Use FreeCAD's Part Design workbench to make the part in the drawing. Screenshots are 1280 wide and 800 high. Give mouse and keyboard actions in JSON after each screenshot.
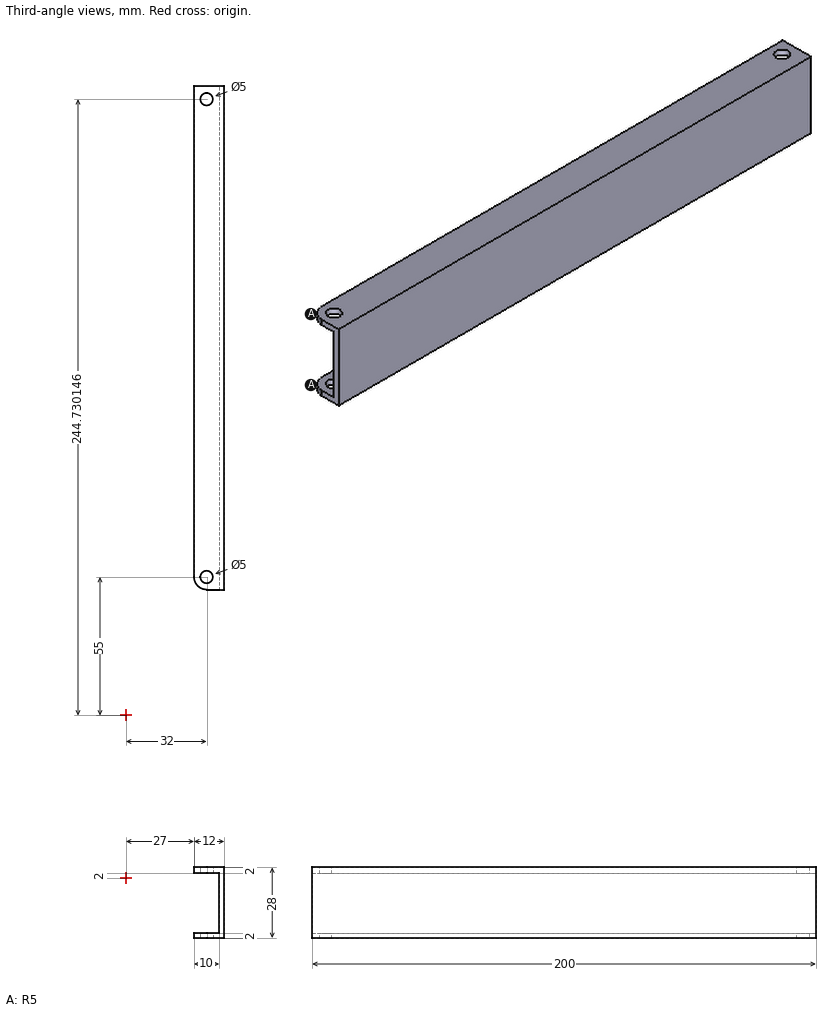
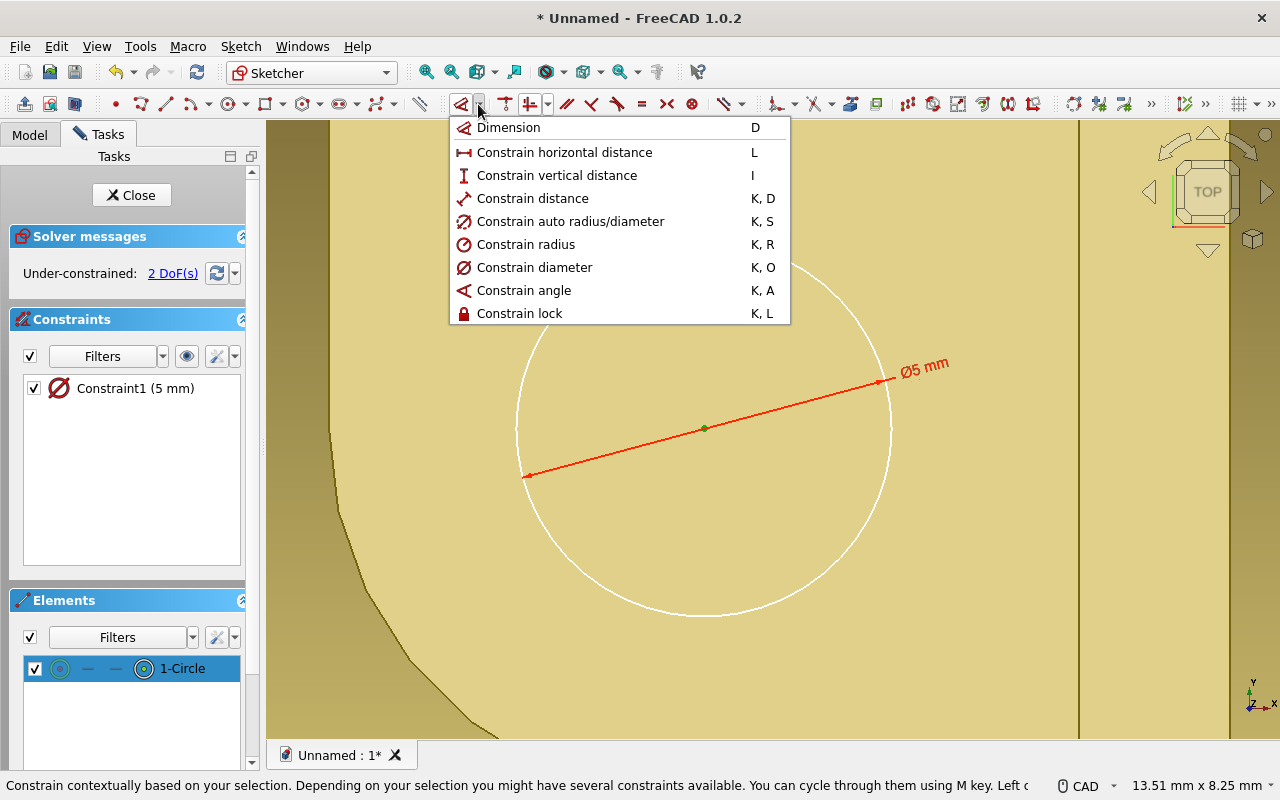
{"action": "left_click", "coordinate": [620, 152]}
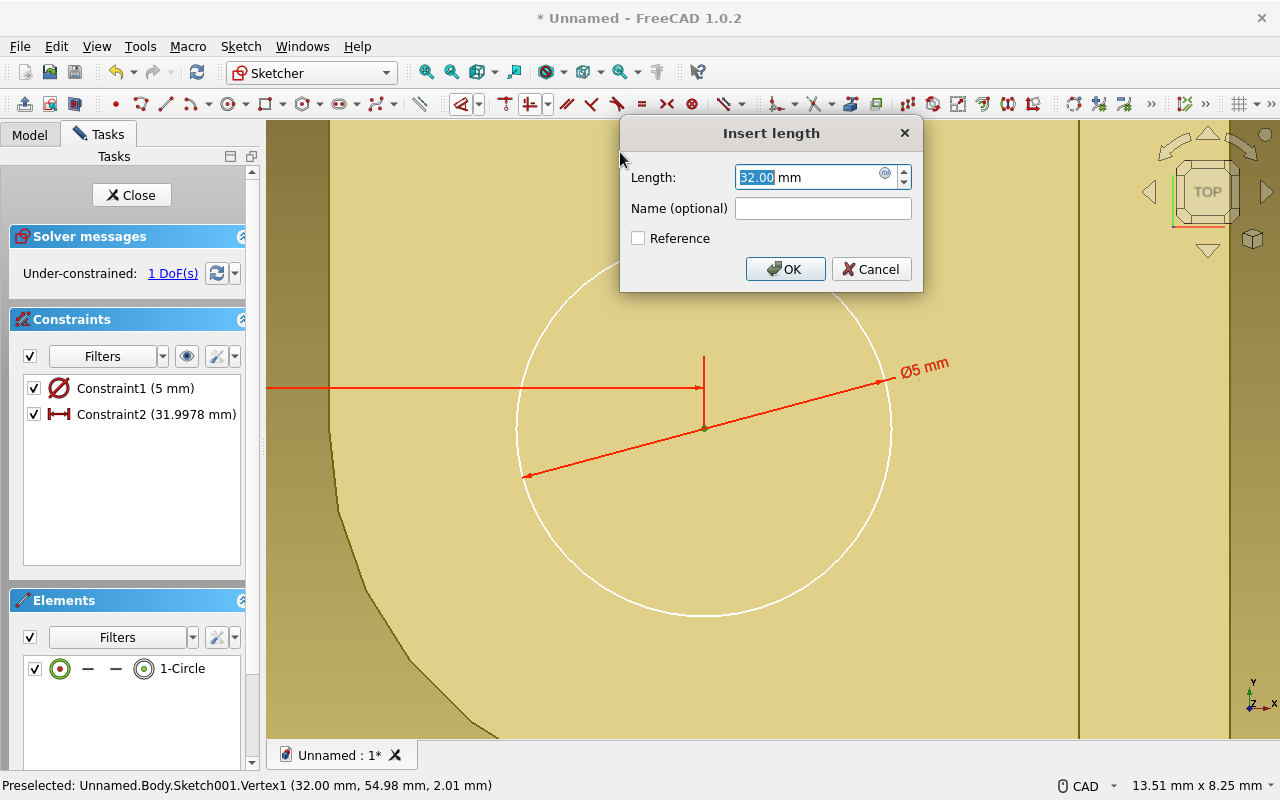
{"action": "type", "text": "32"}
{"action": "key", "text": "Return"}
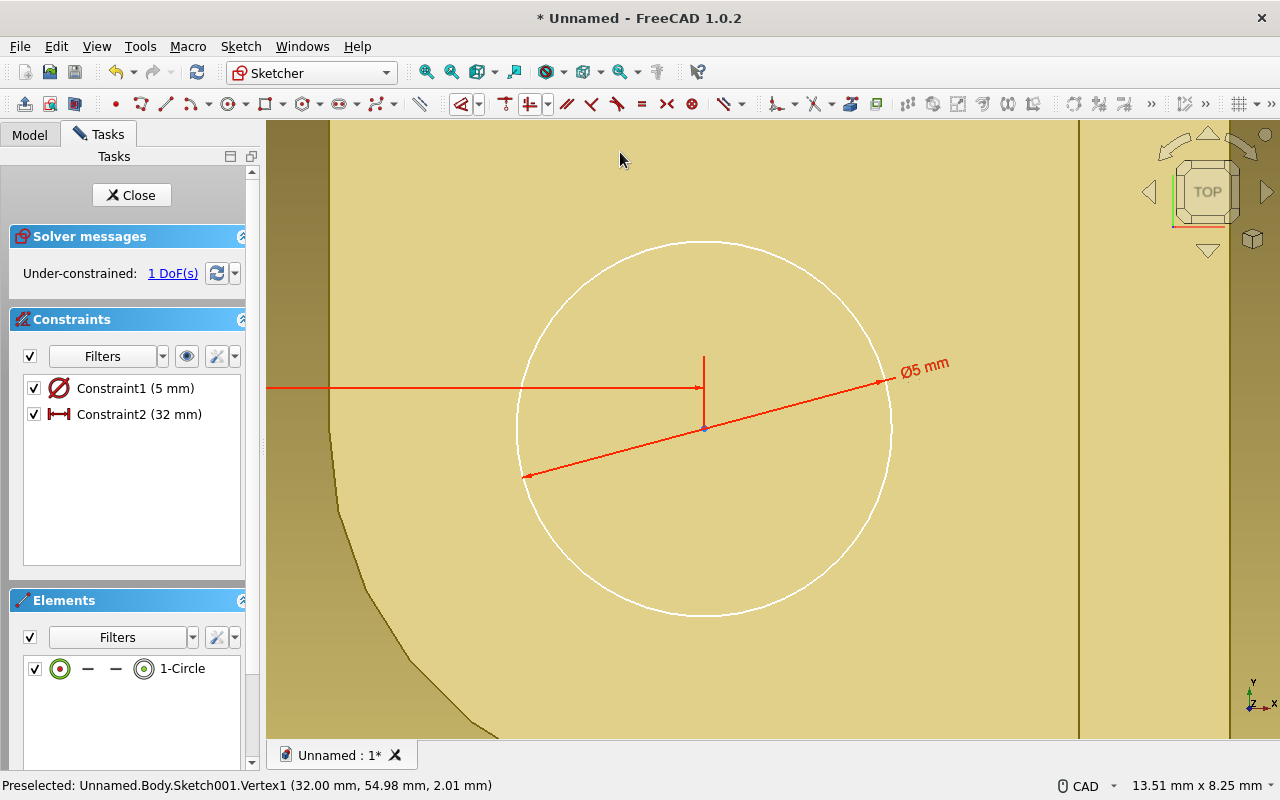
{"action": "left_click", "coordinate": [704, 429]}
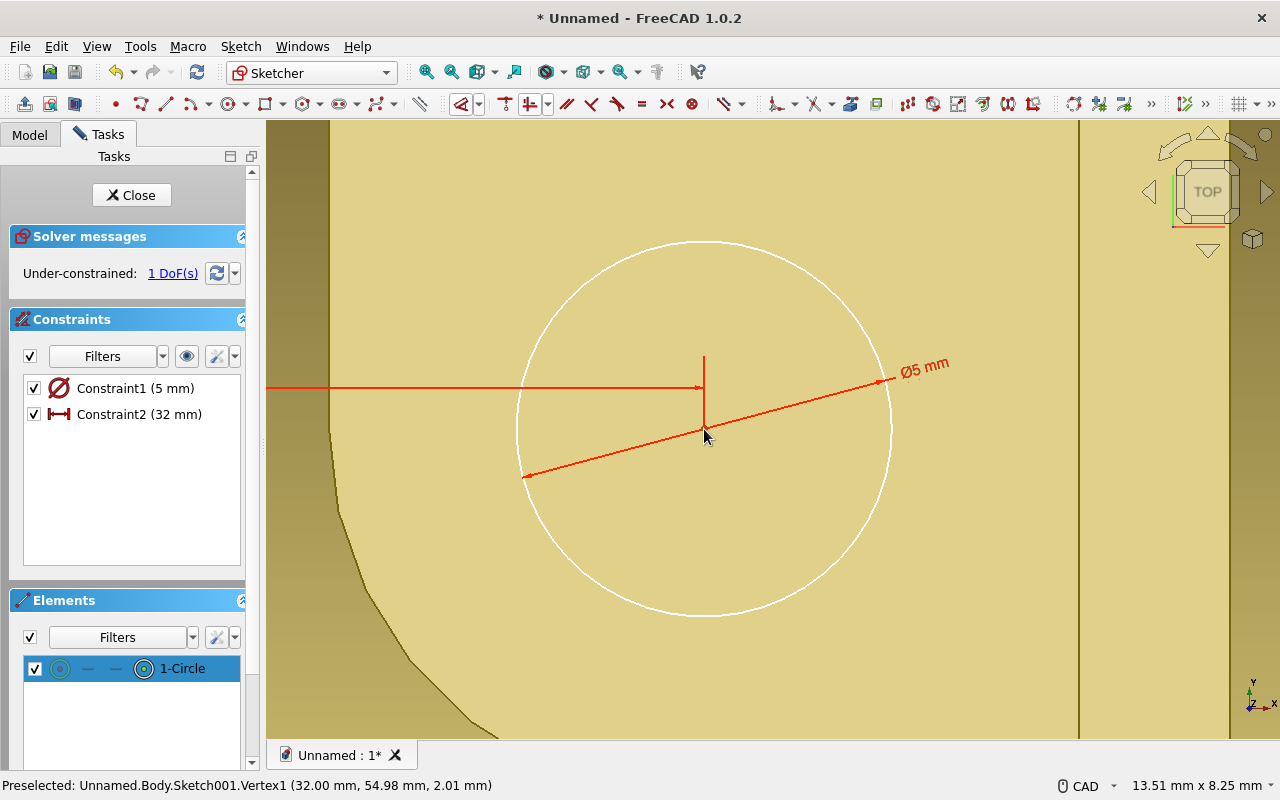
{"action": "key", "text": "i"}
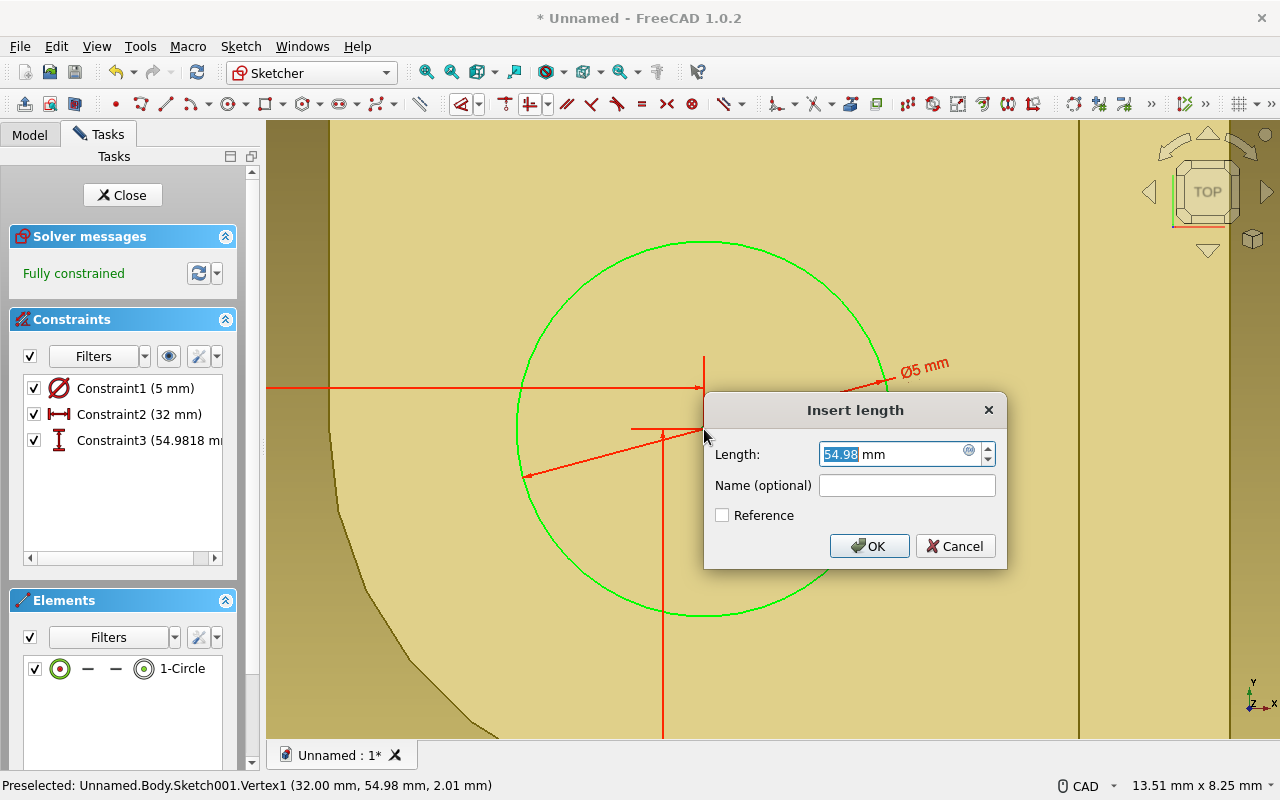
{"action": "type", "text": "55"}
{"action": "key", "text": "Return"}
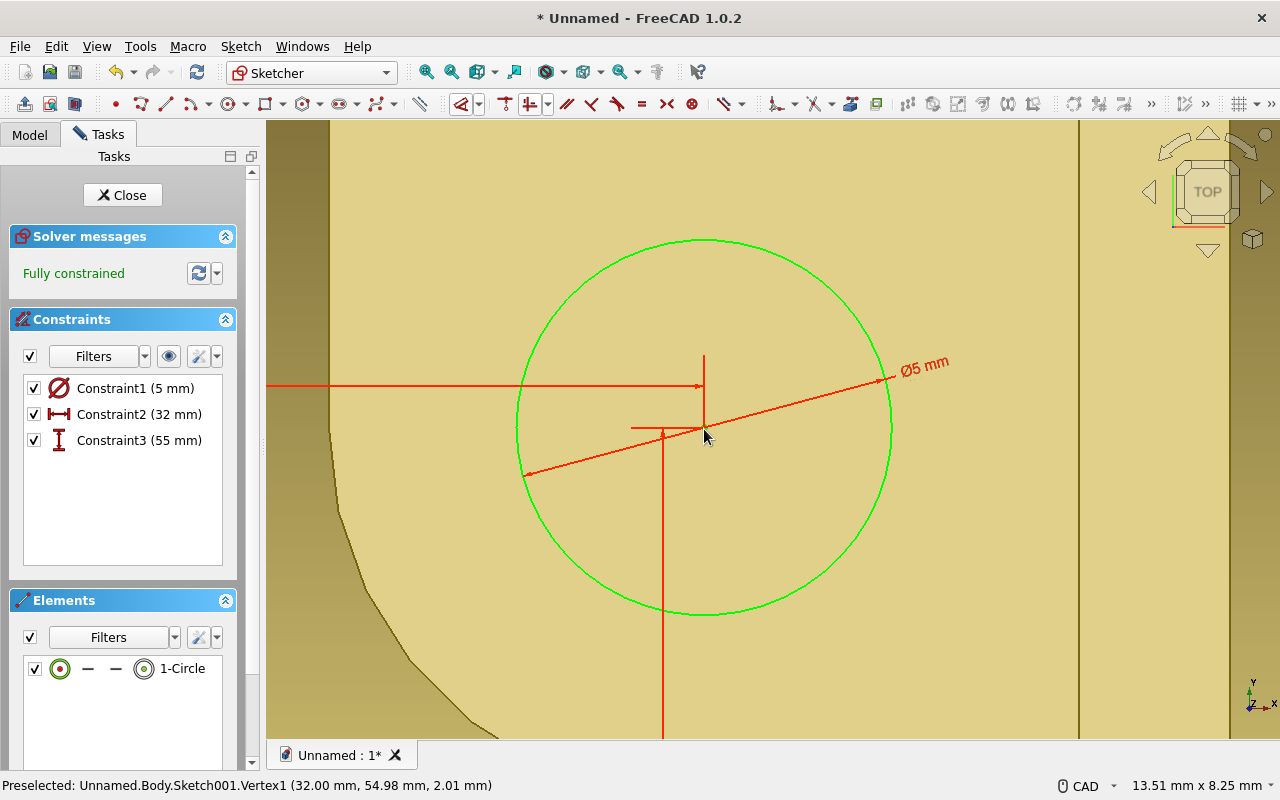
{"action": "left_click", "coordinate": [123, 195]}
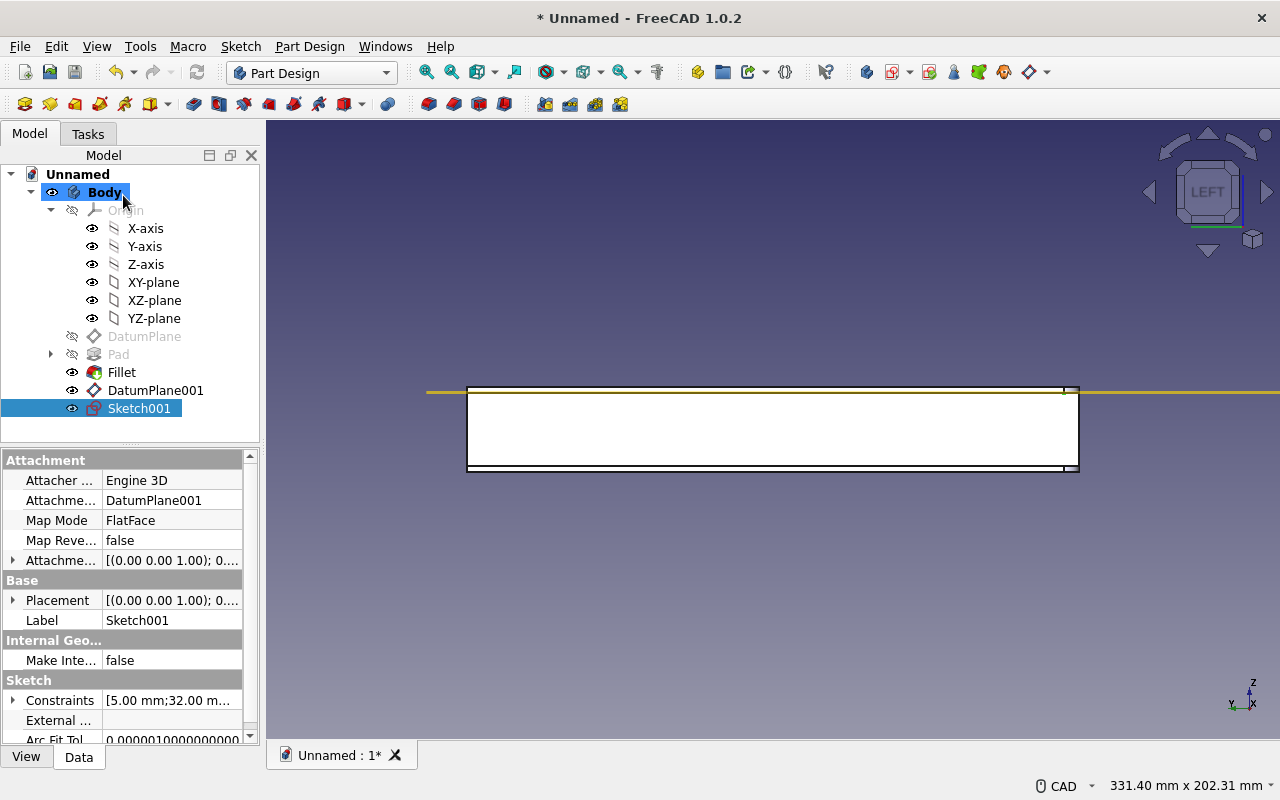
{"action": "left_click", "coordinate": [194, 104]}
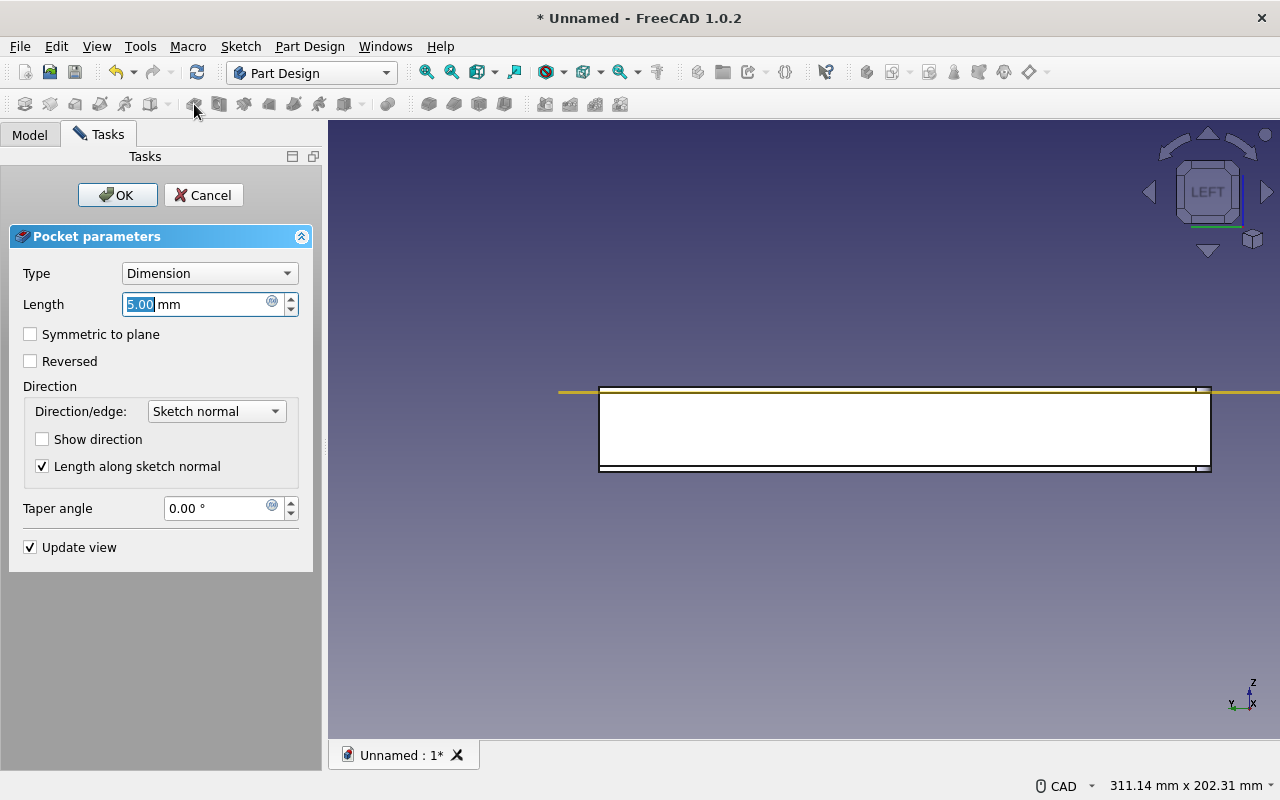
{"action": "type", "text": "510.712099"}
{"action": "key", "text": "Tab"}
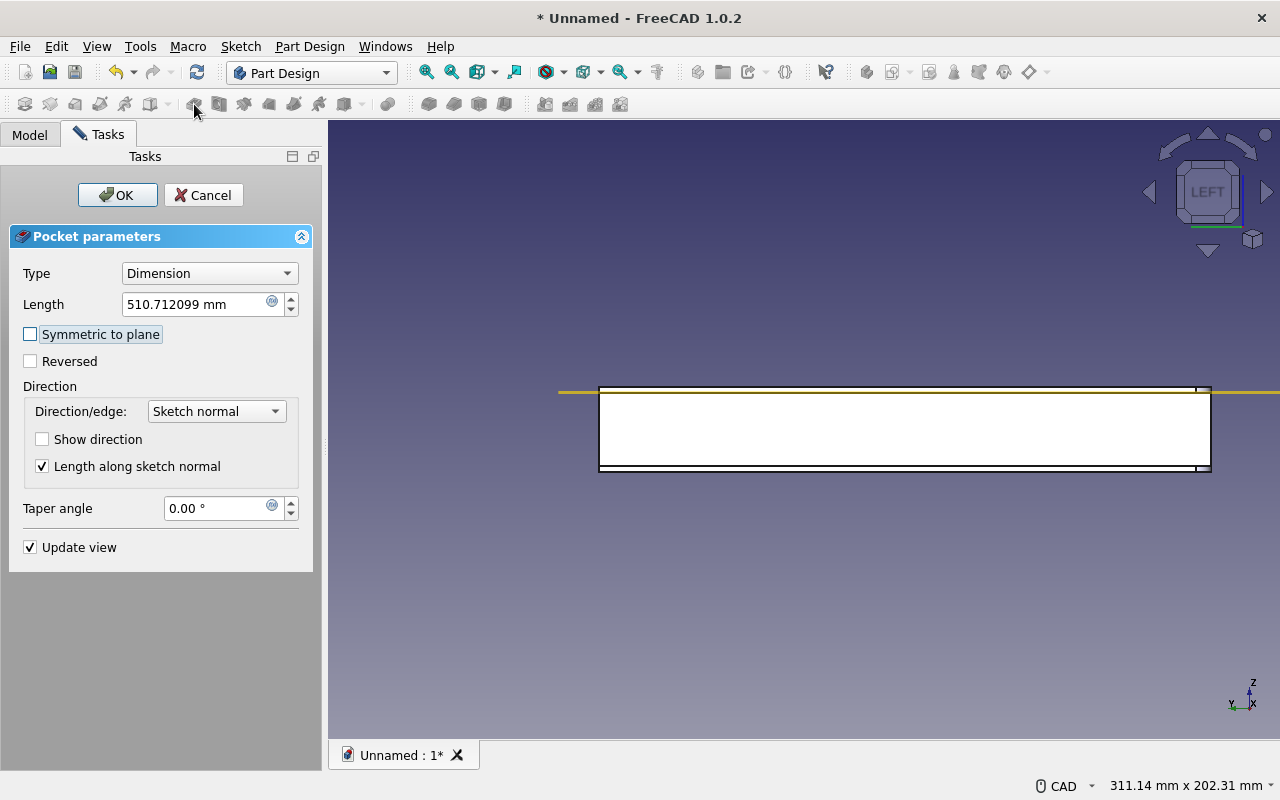
{"action": "left_click", "coordinate": [31, 334]}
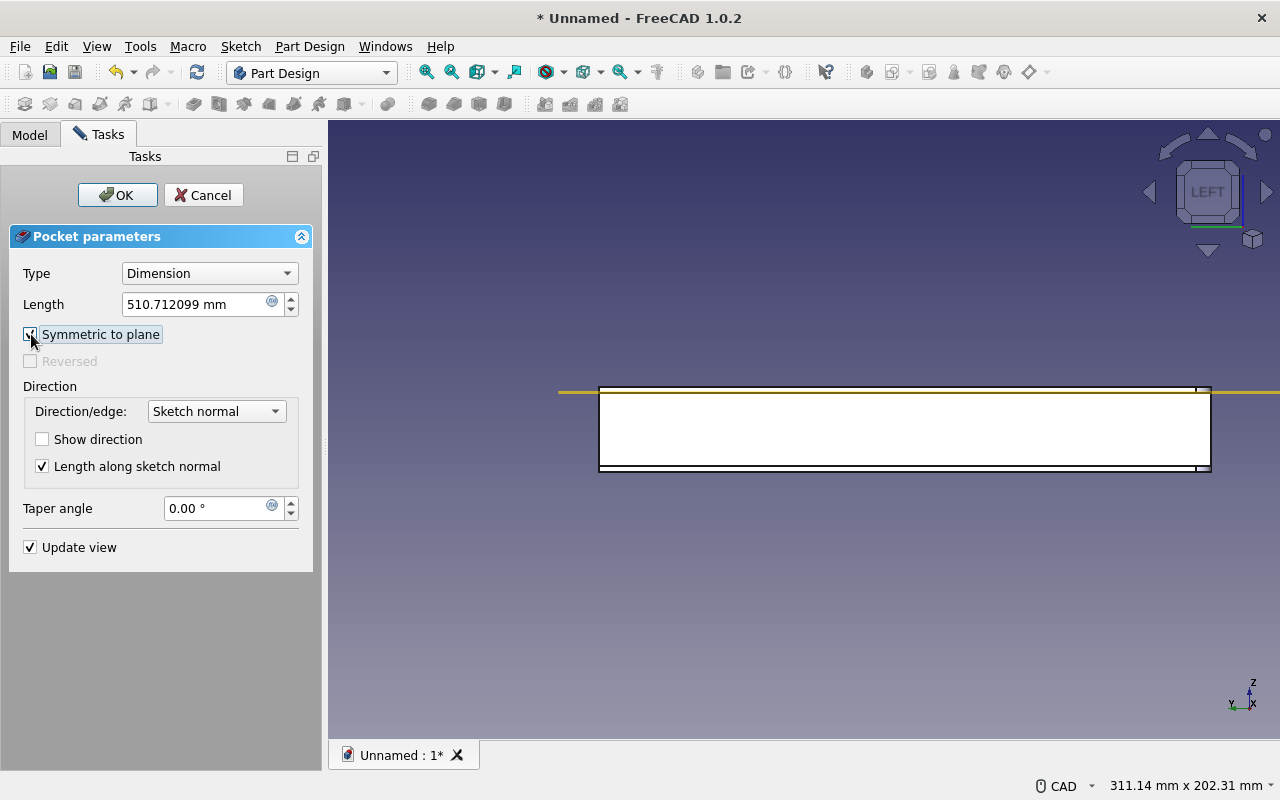
{"action": "left_click", "coordinate": [118, 195]}